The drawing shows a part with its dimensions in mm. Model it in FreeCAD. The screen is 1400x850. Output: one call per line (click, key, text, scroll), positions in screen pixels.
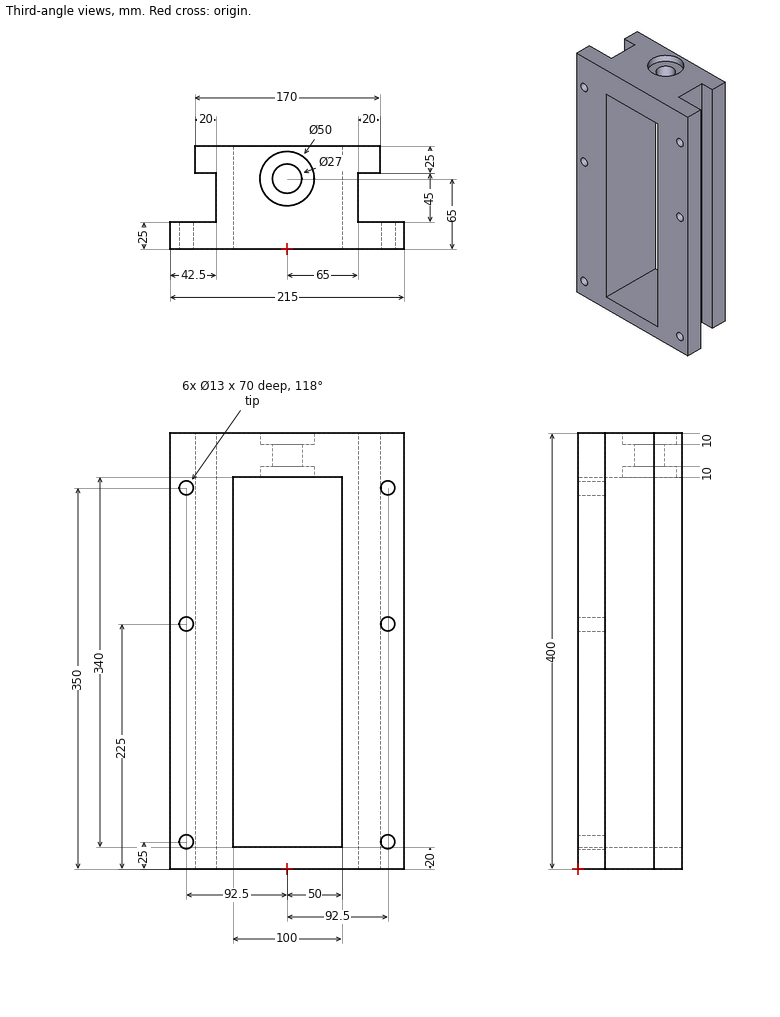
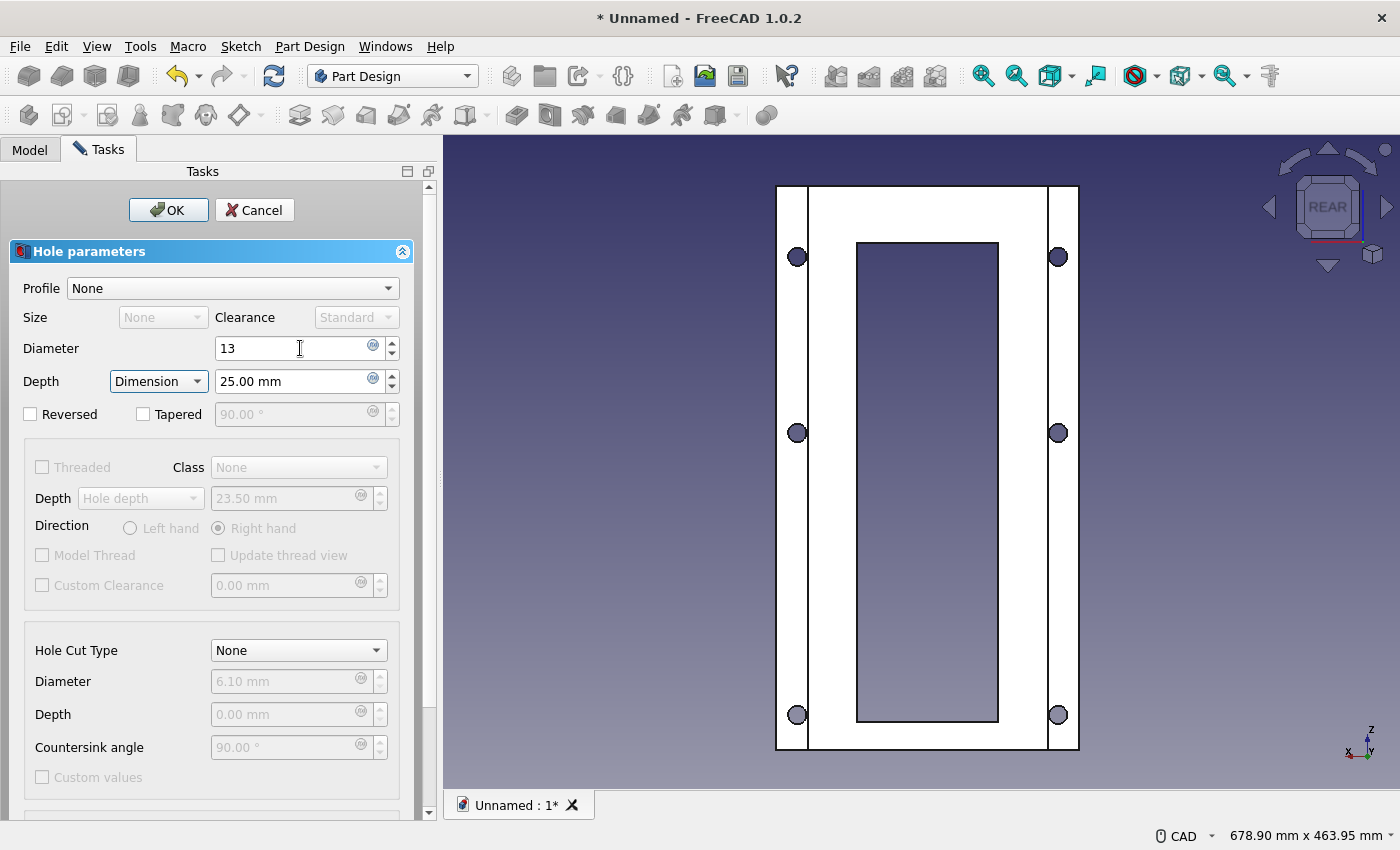
triple_click(300, 382)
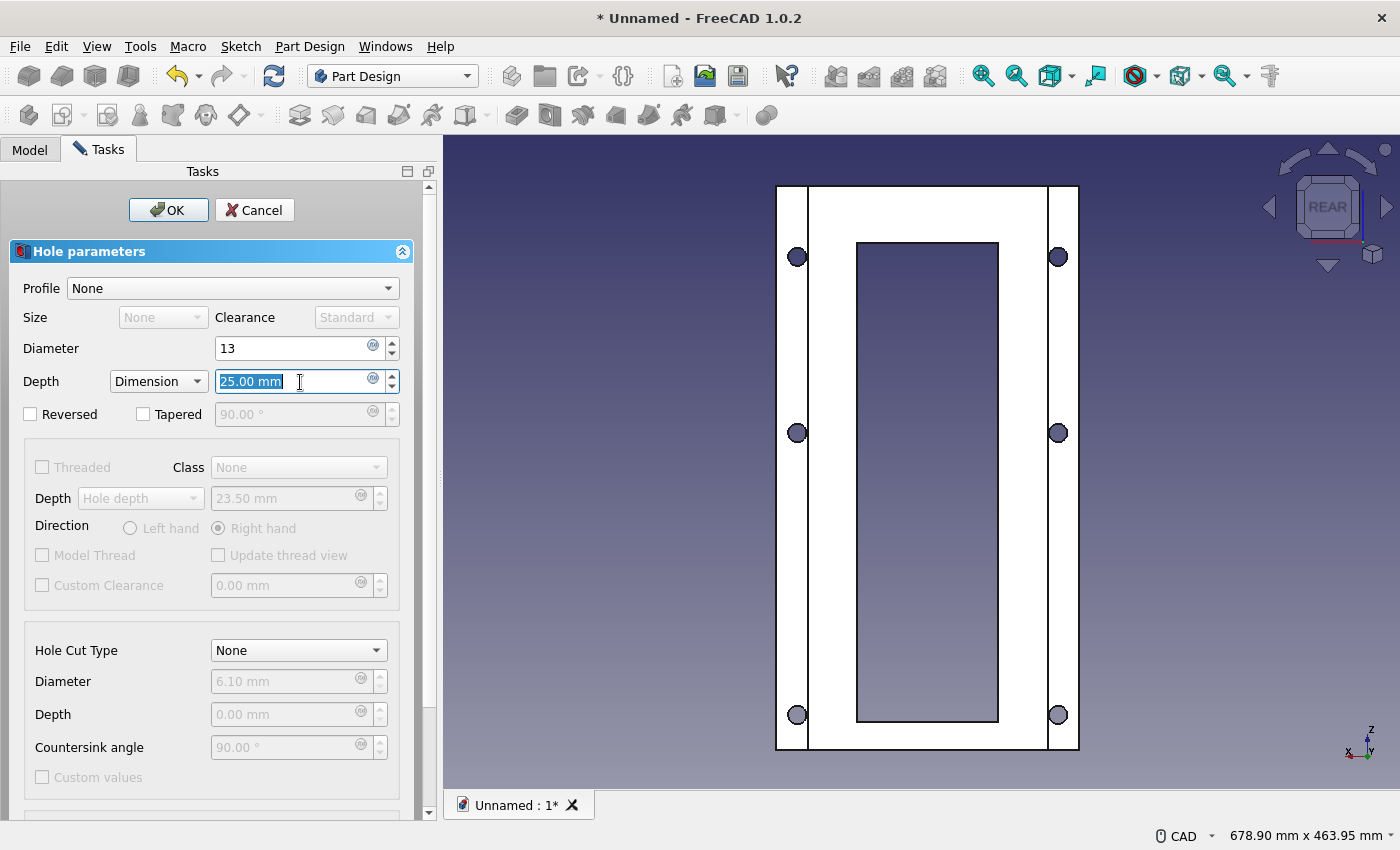
text(70)
key(Tab)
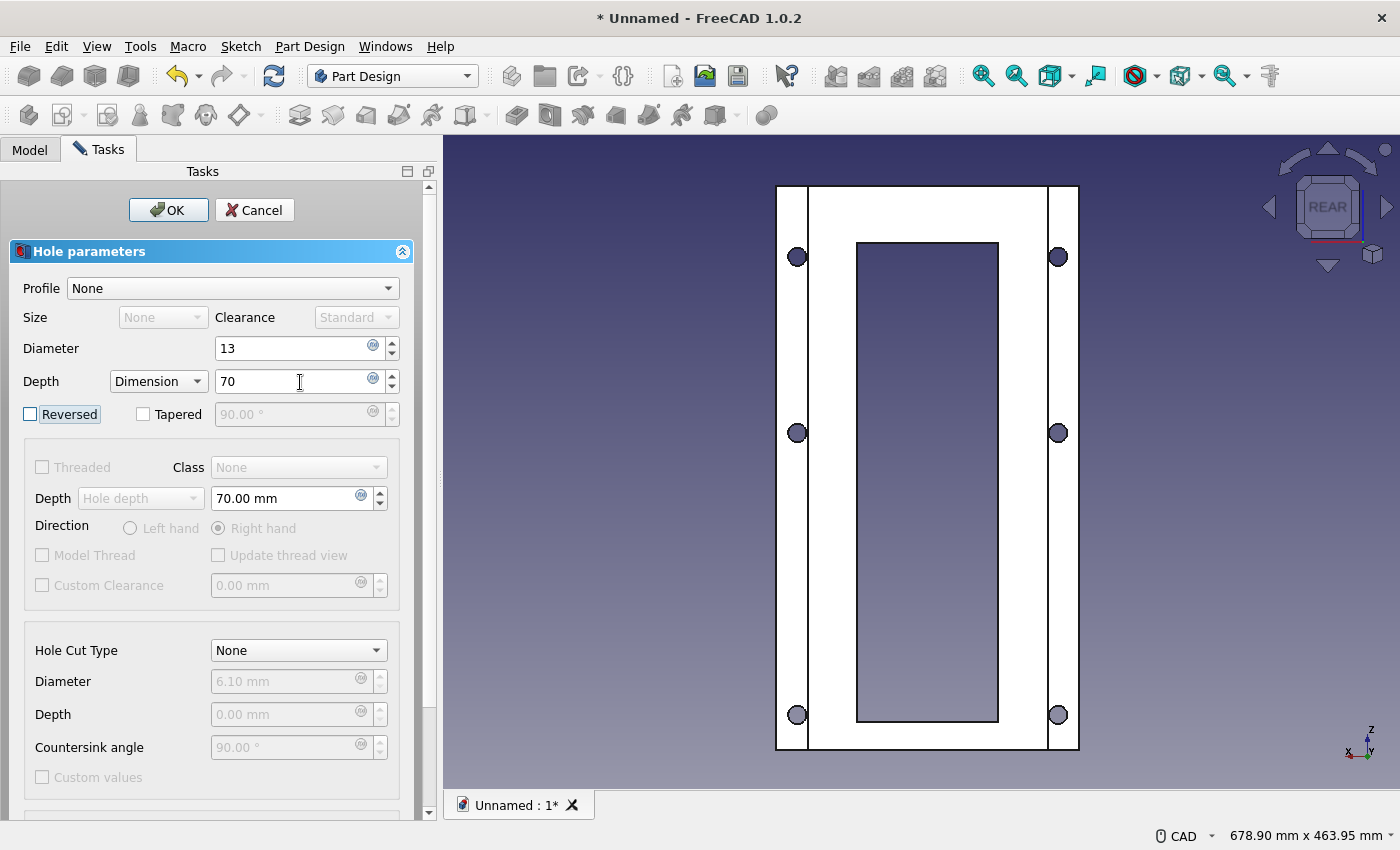
click(169, 210)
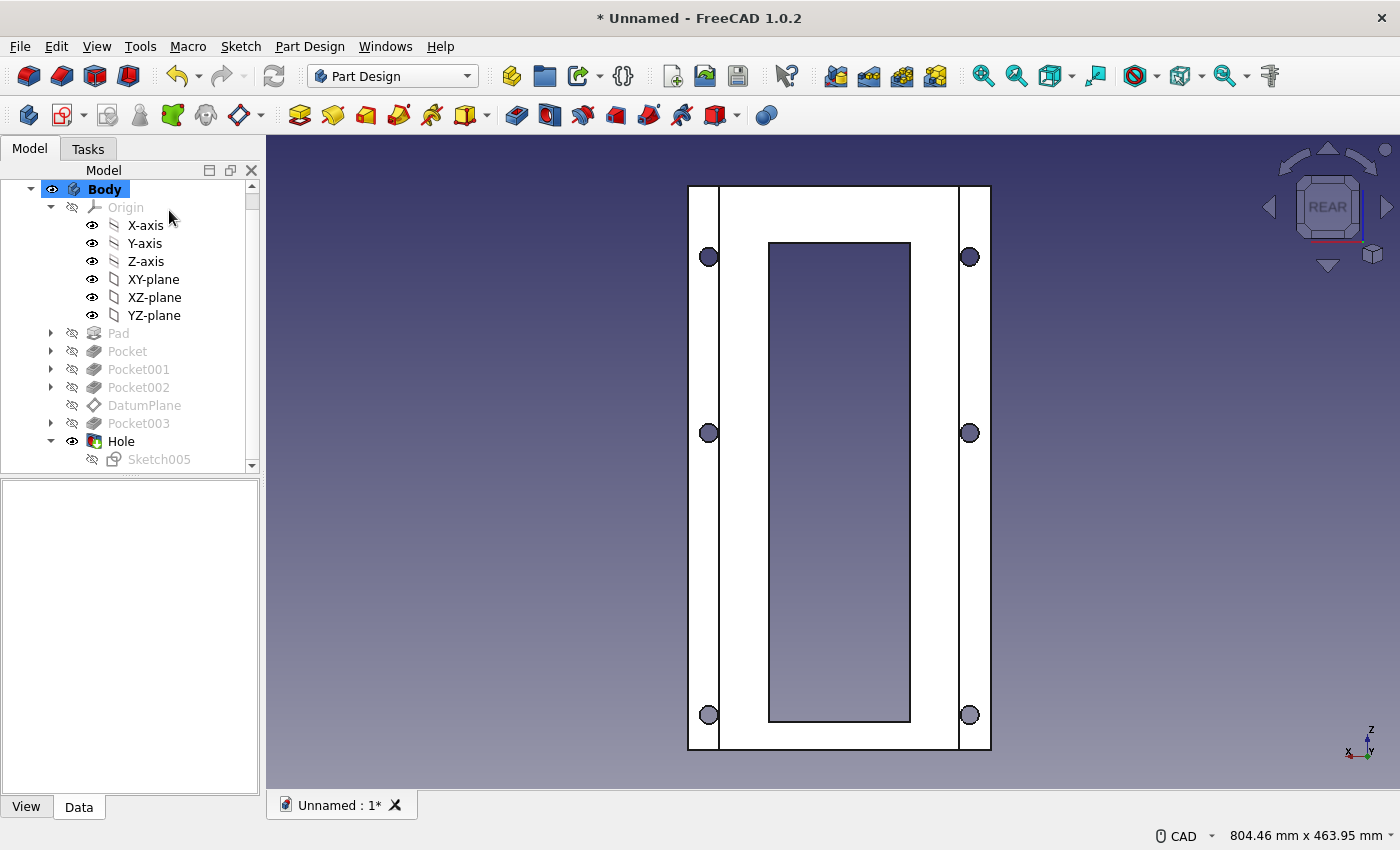
key(0)